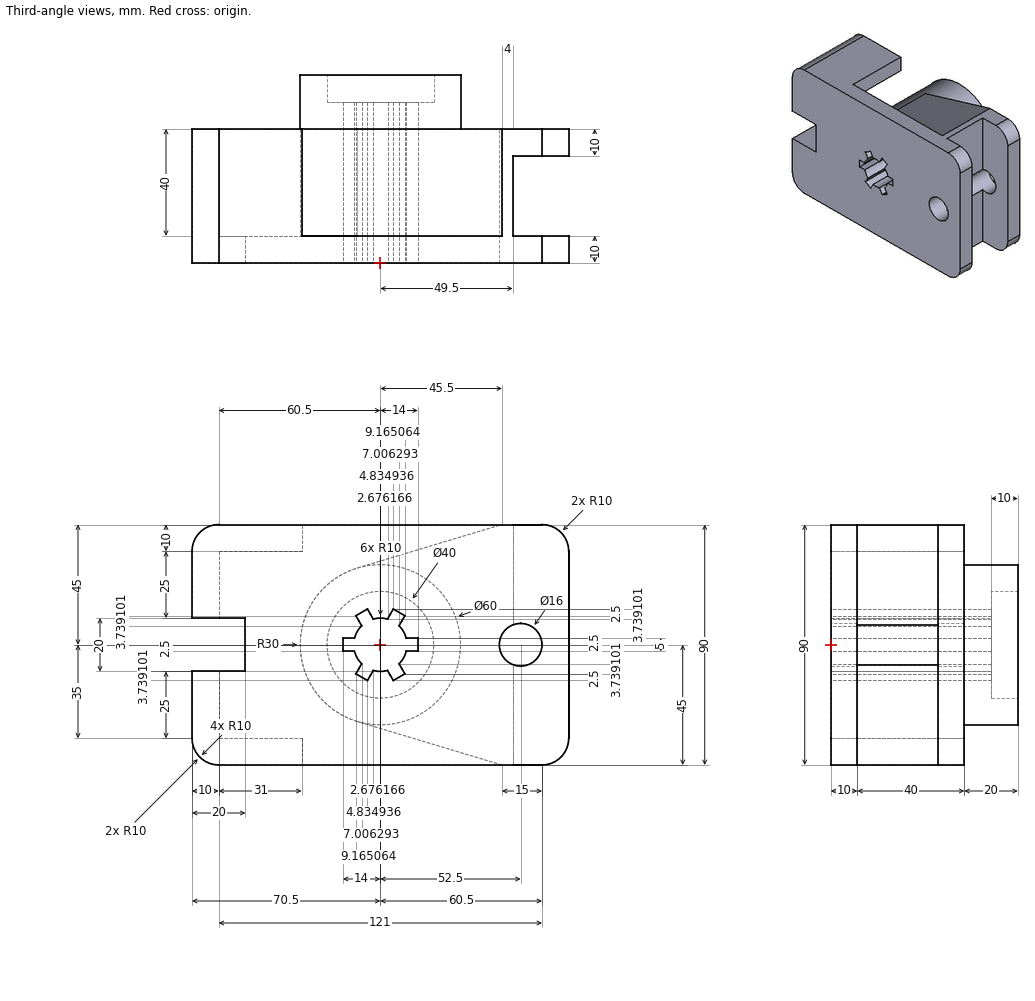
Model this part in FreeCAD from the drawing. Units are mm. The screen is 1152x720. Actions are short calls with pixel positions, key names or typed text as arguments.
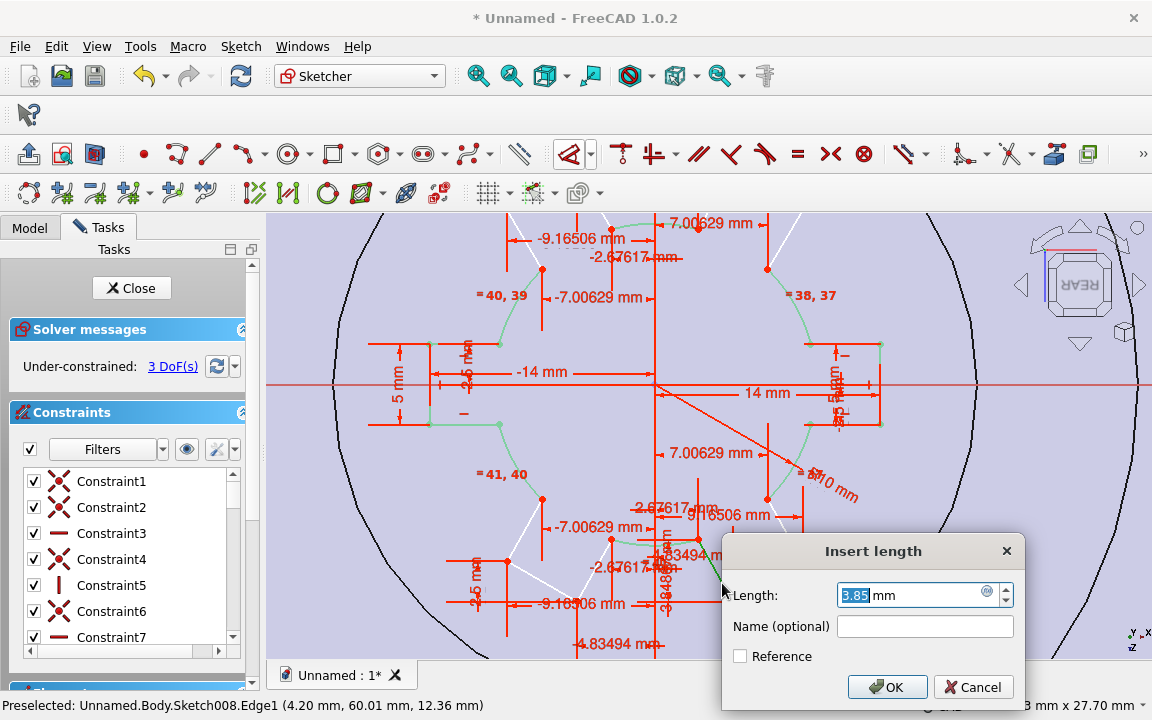
text(3.739101)
key(Return)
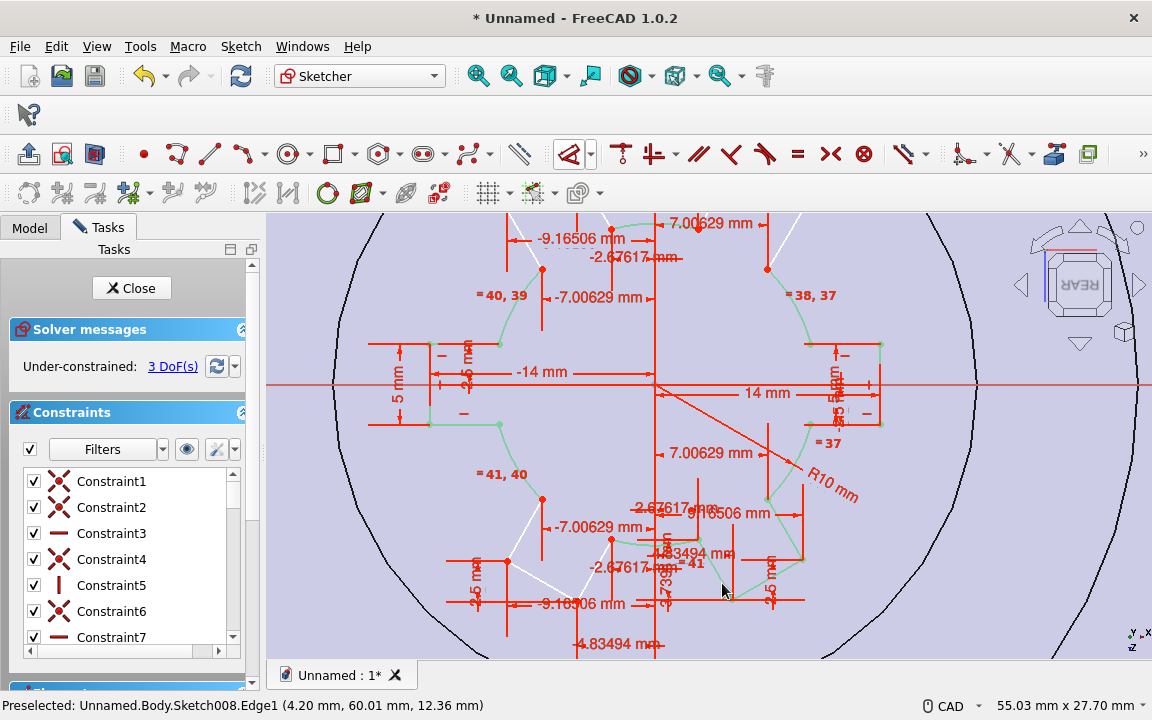
click(778, 252)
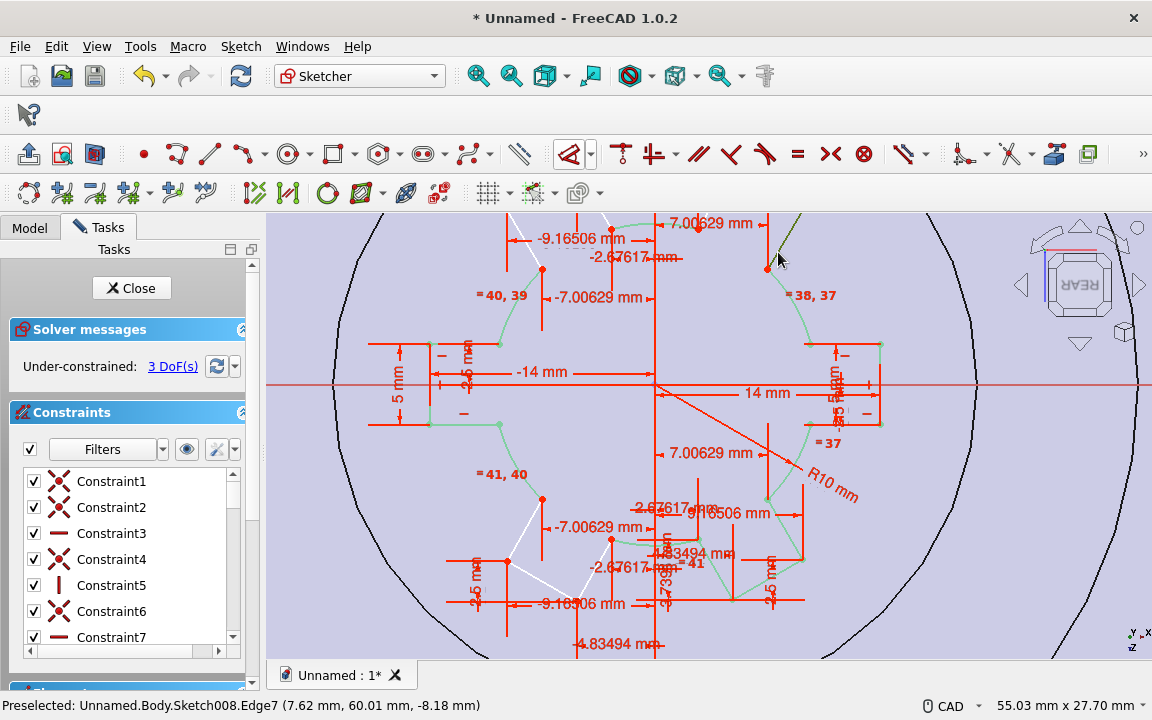
click(590, 154)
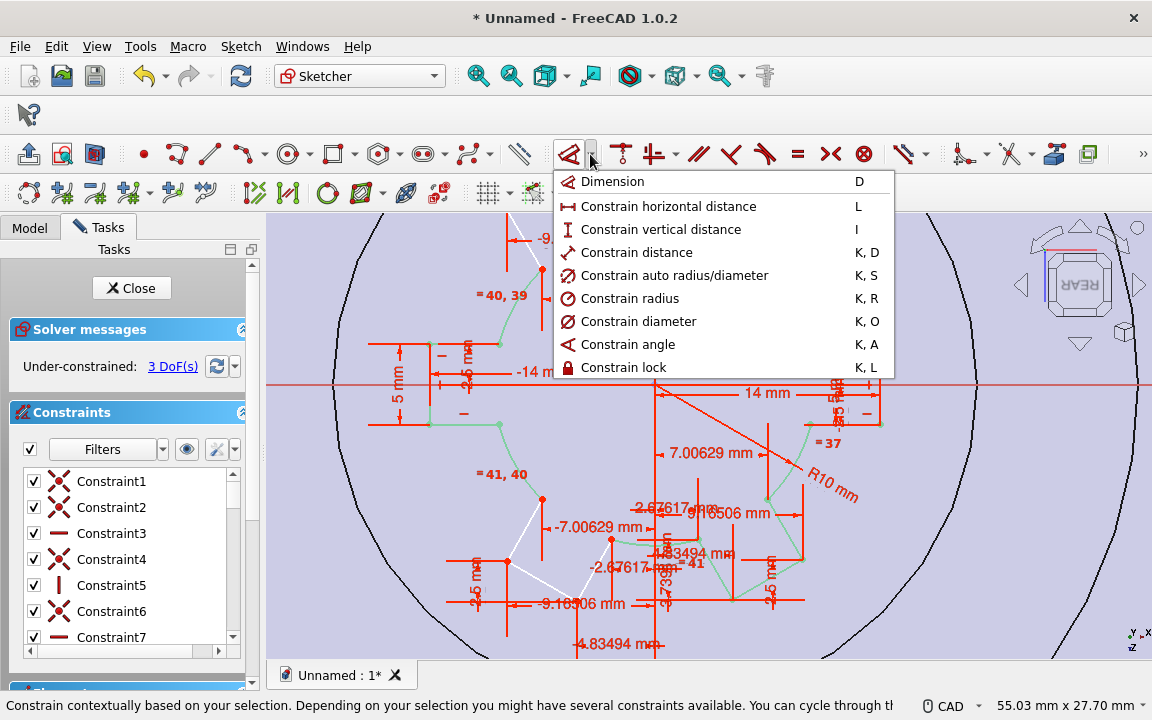
click(724, 230)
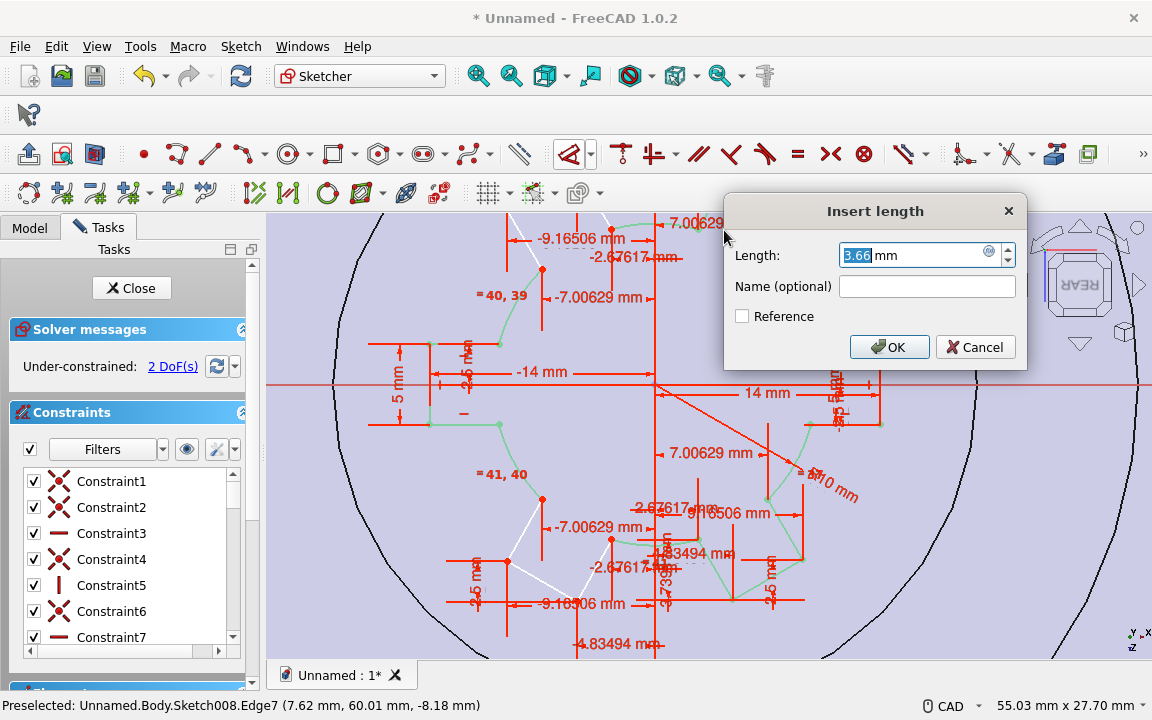
text(3.739101)
key(Return)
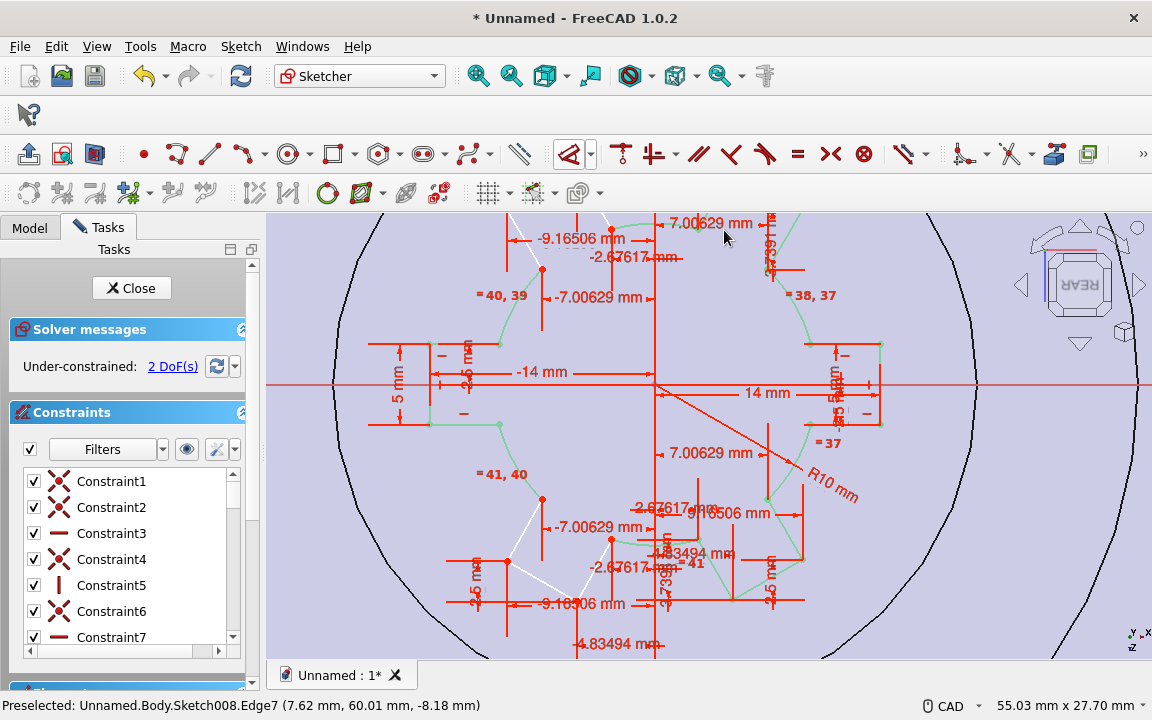
scroll(611, 541, down, 2)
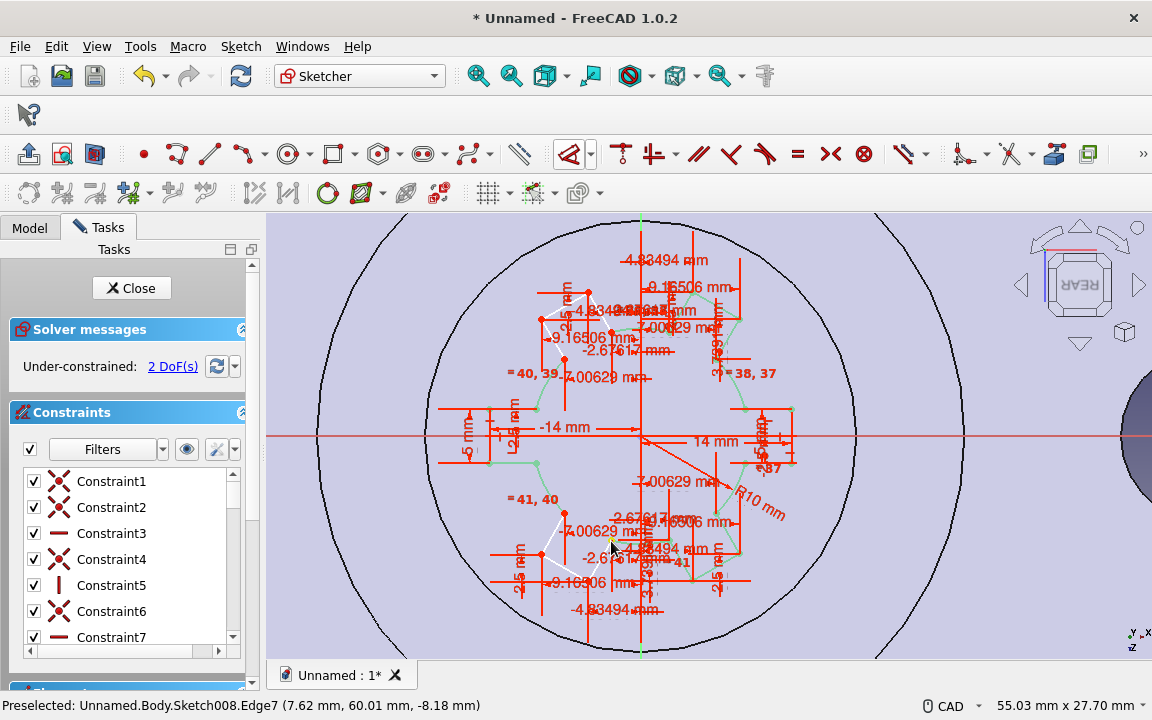
click(605, 321)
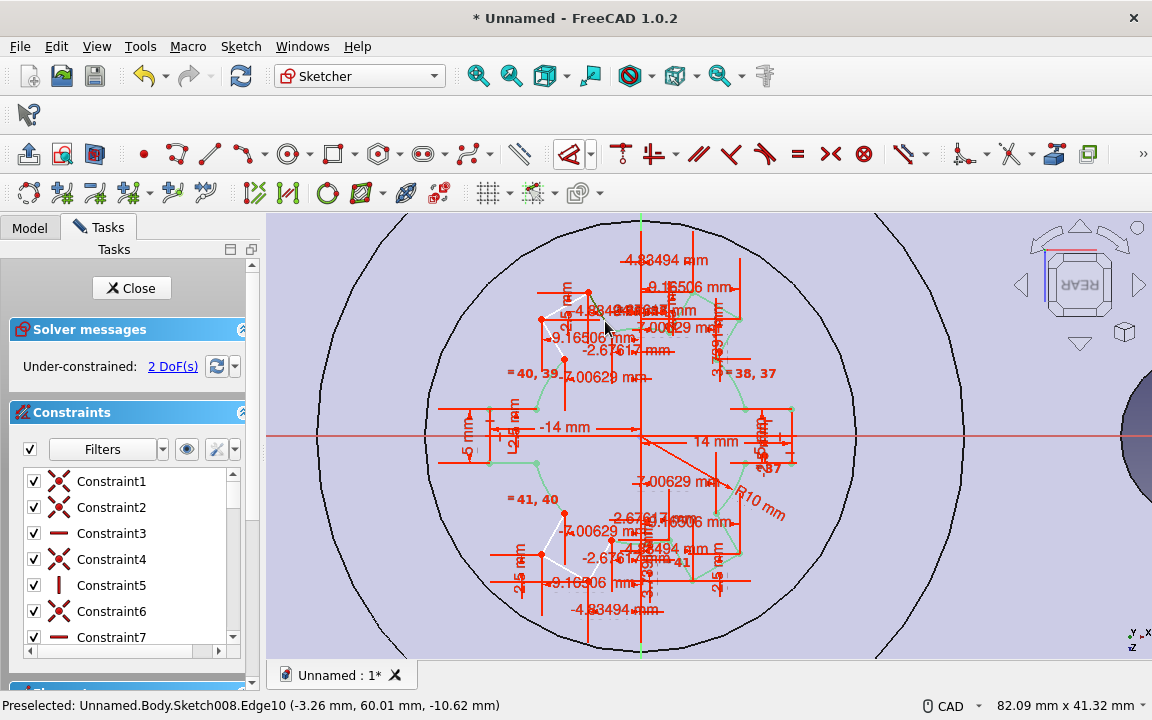
click(590, 154)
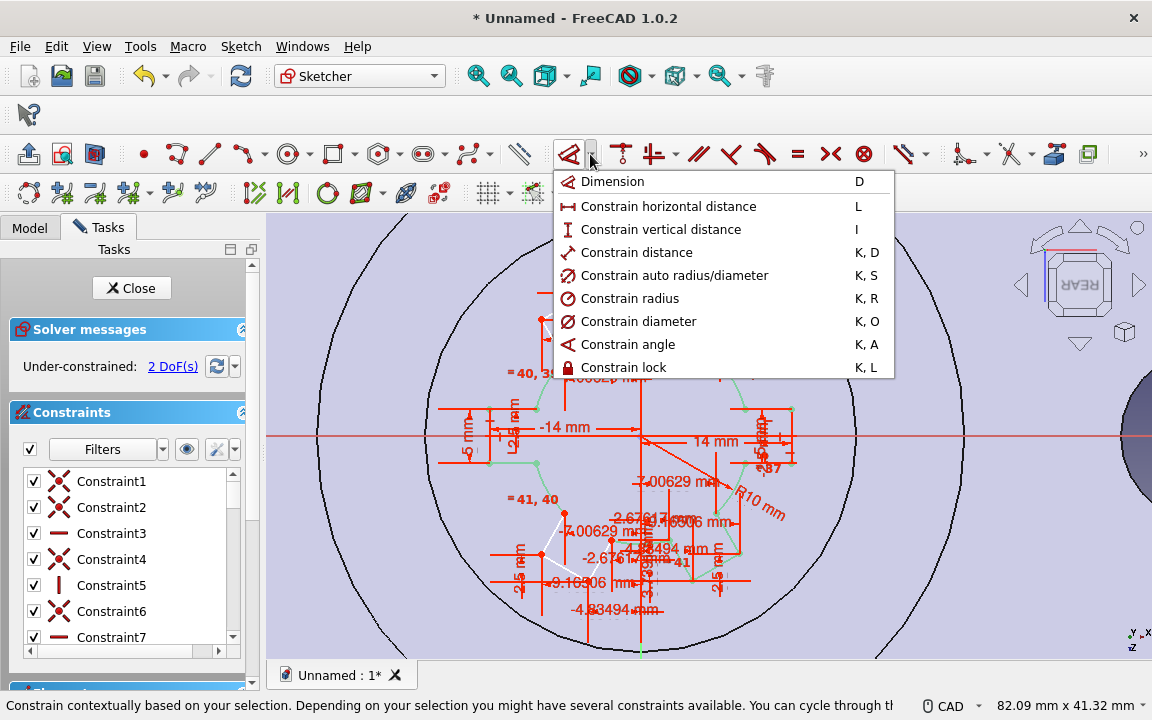
click(724, 230)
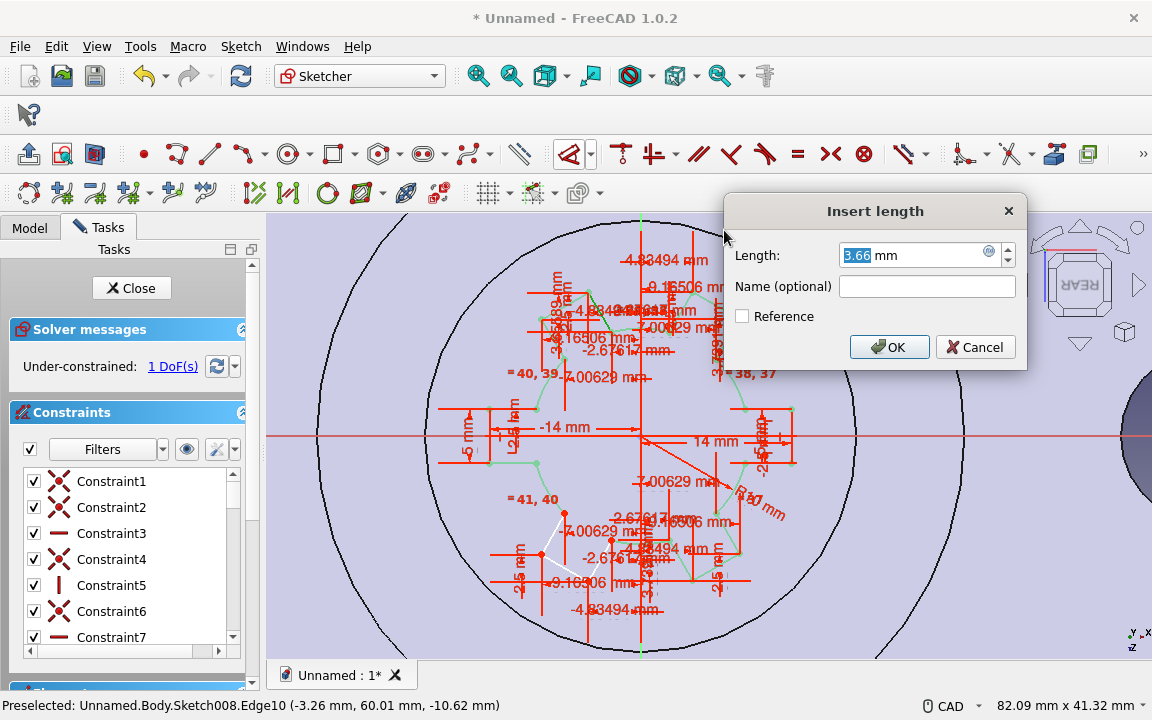
text(3.739101)
key(Return)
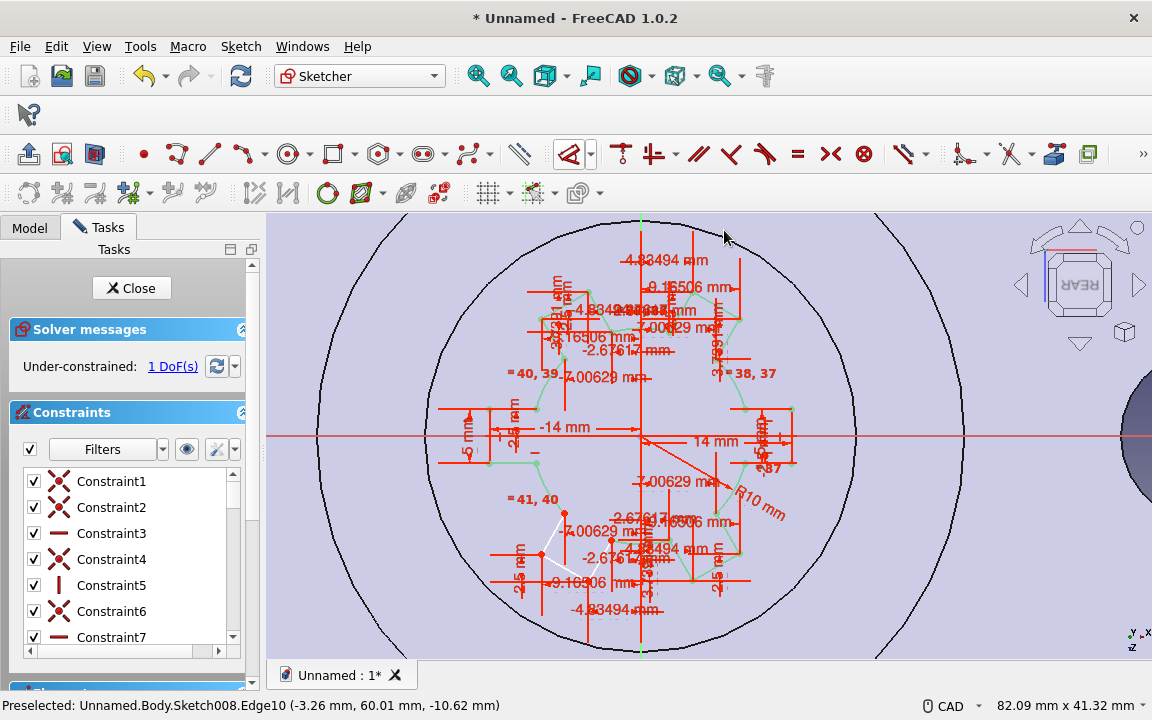
click(558, 526)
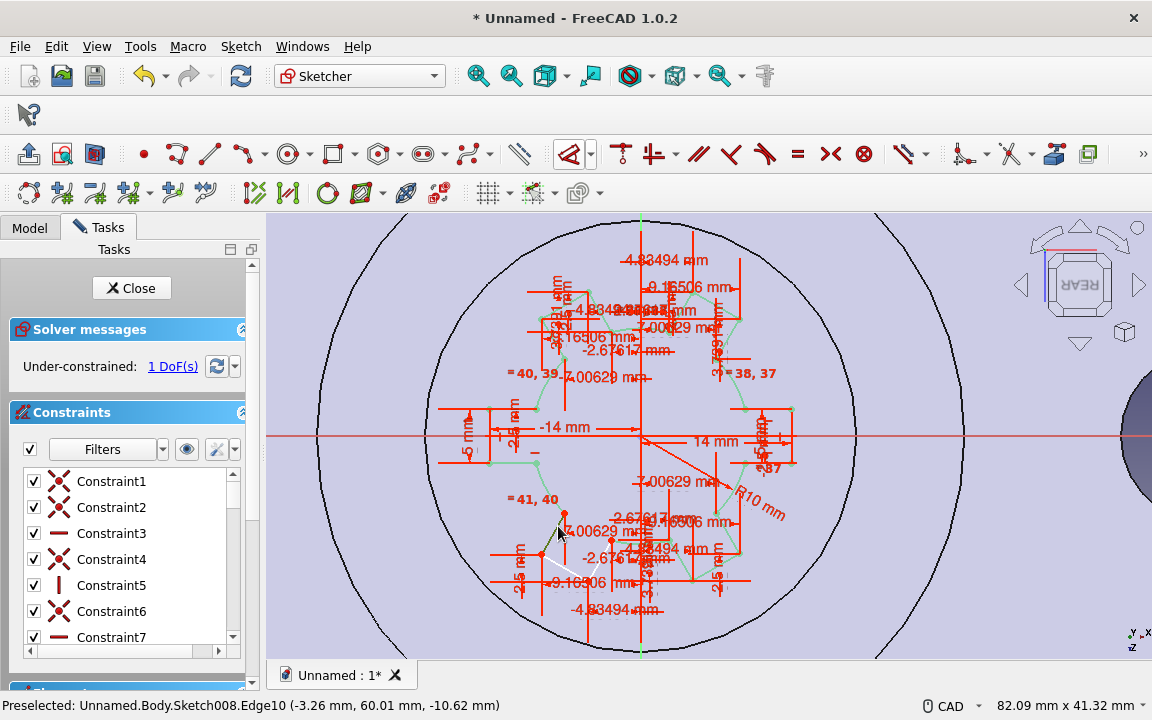
click(590, 154)